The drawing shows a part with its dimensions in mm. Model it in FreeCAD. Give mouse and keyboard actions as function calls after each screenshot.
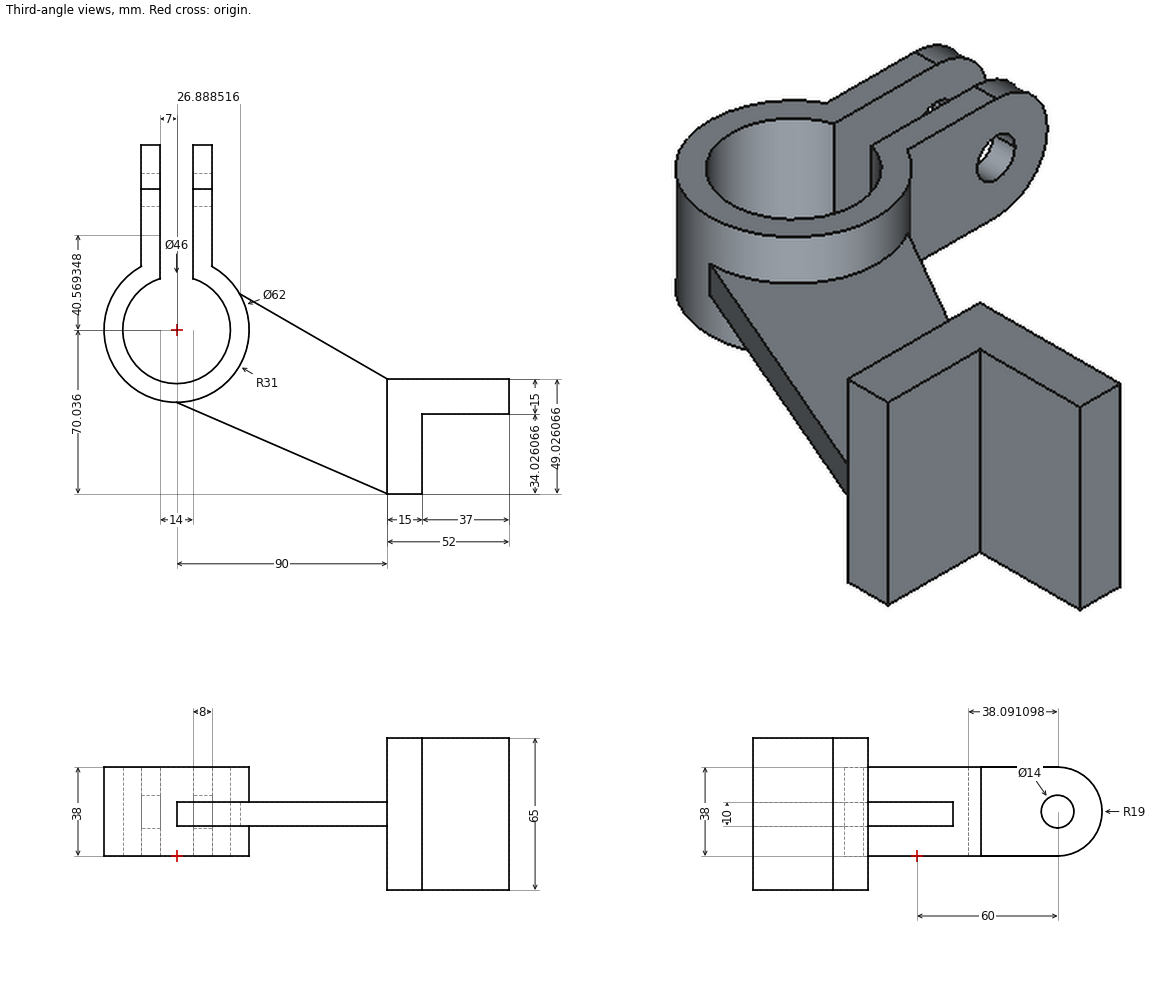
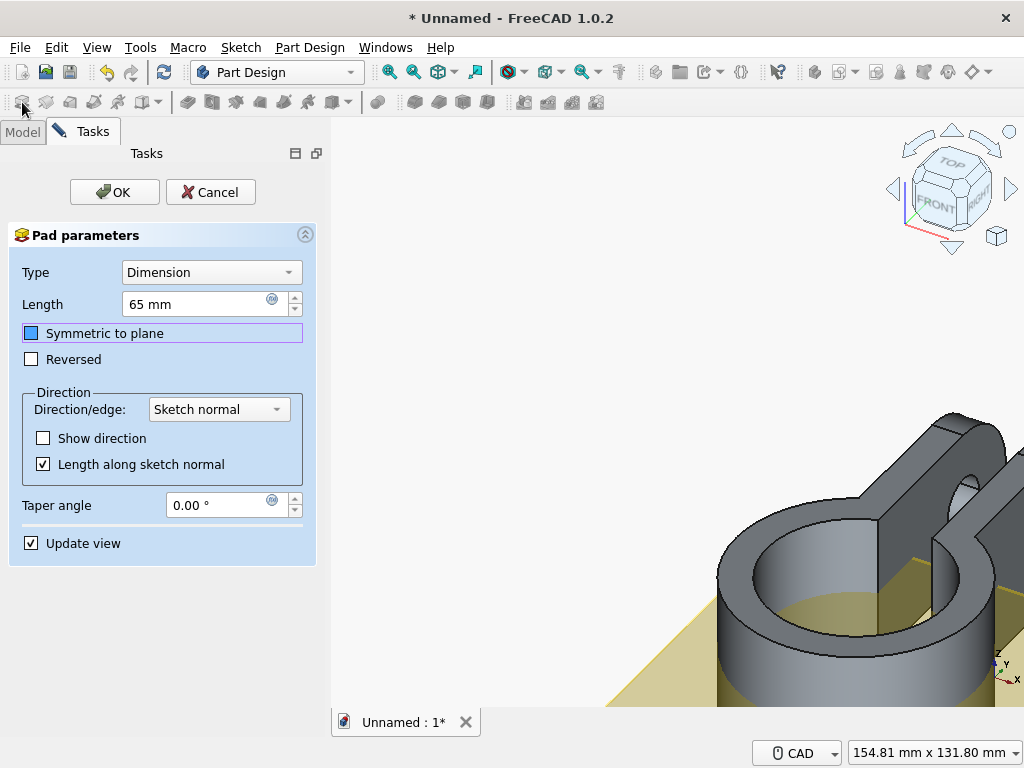
click(30, 333)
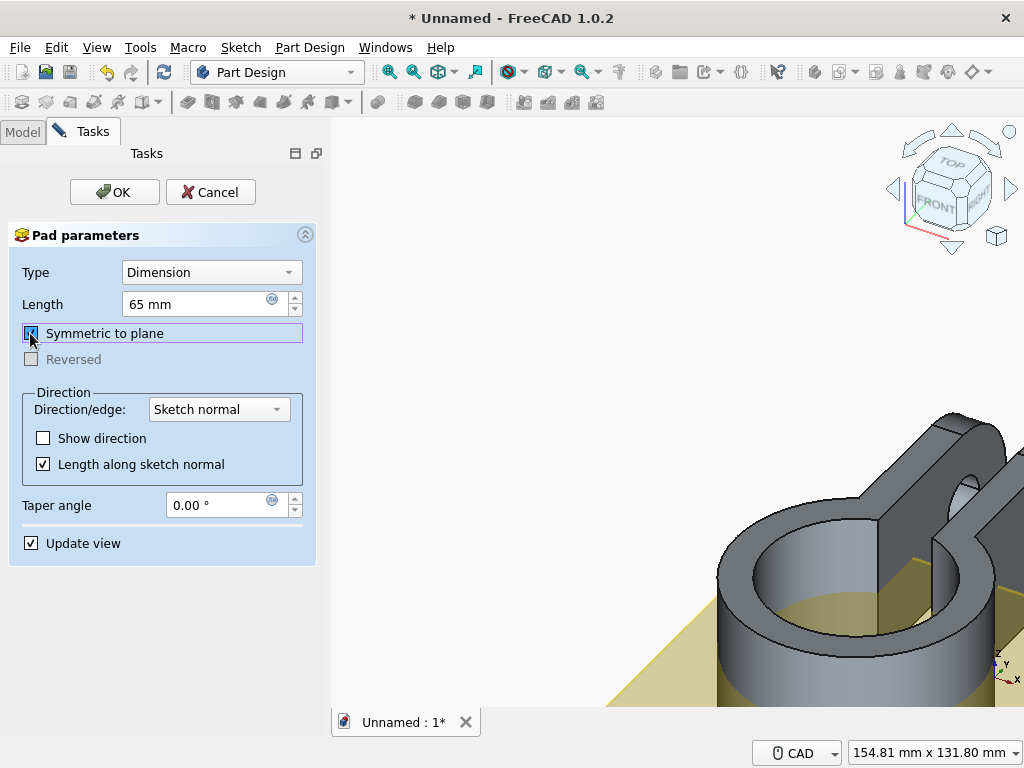
click(115, 192)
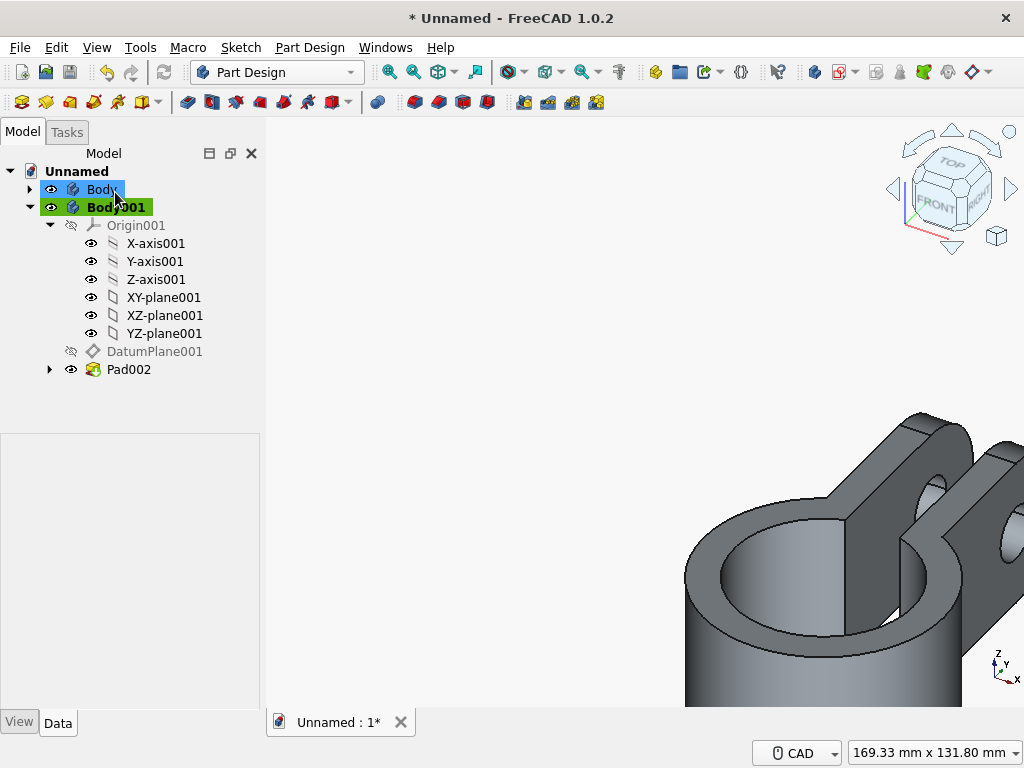
click(390, 72)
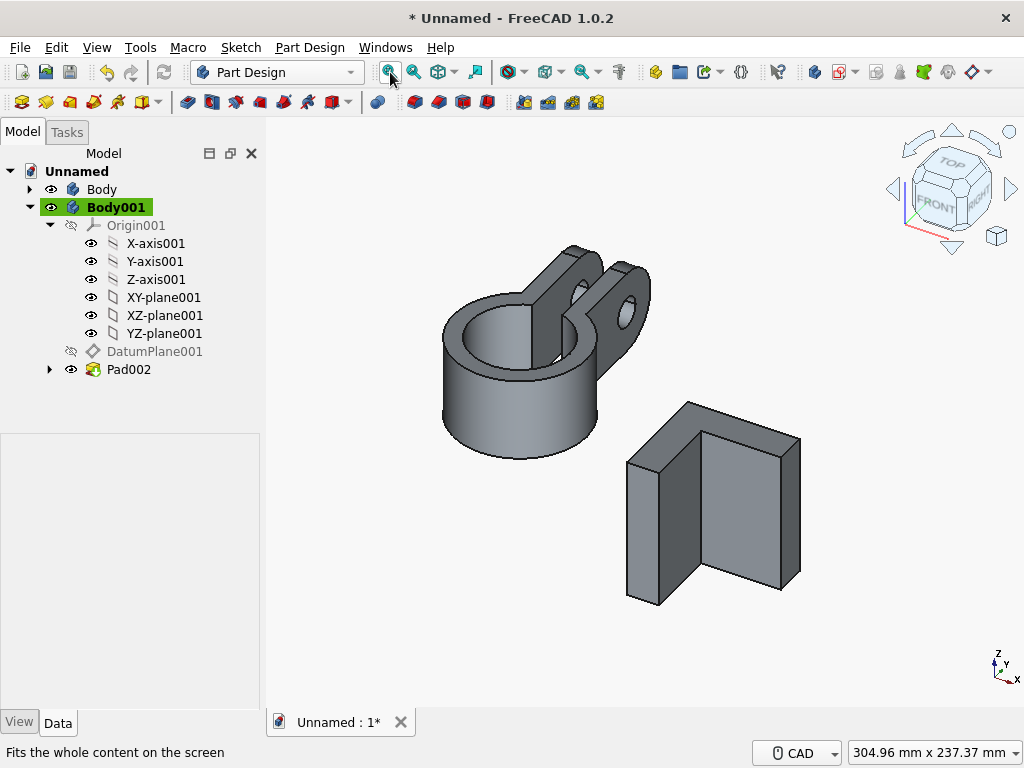
double_click(96, 189)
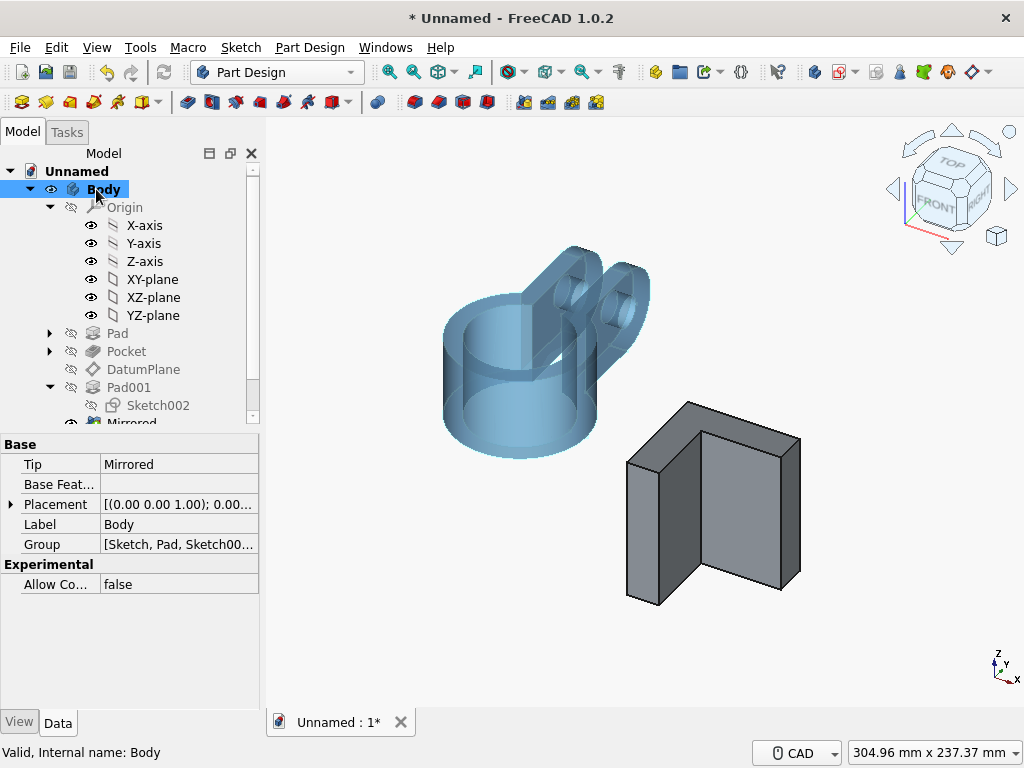
click(96, 189)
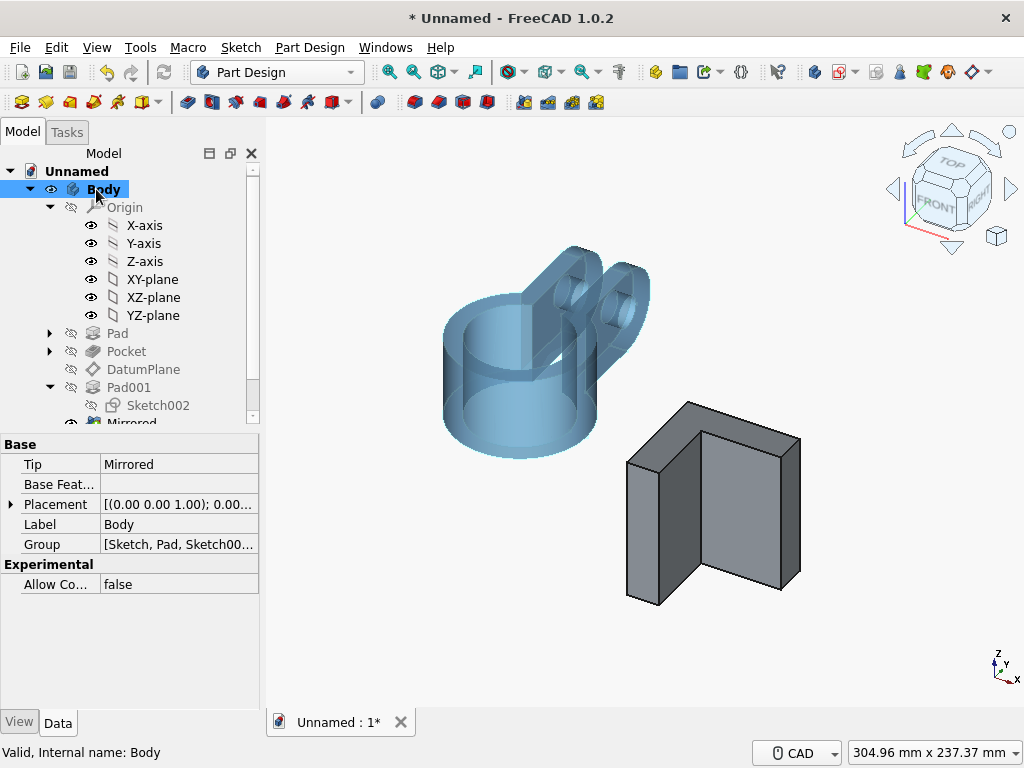
click(146, 584)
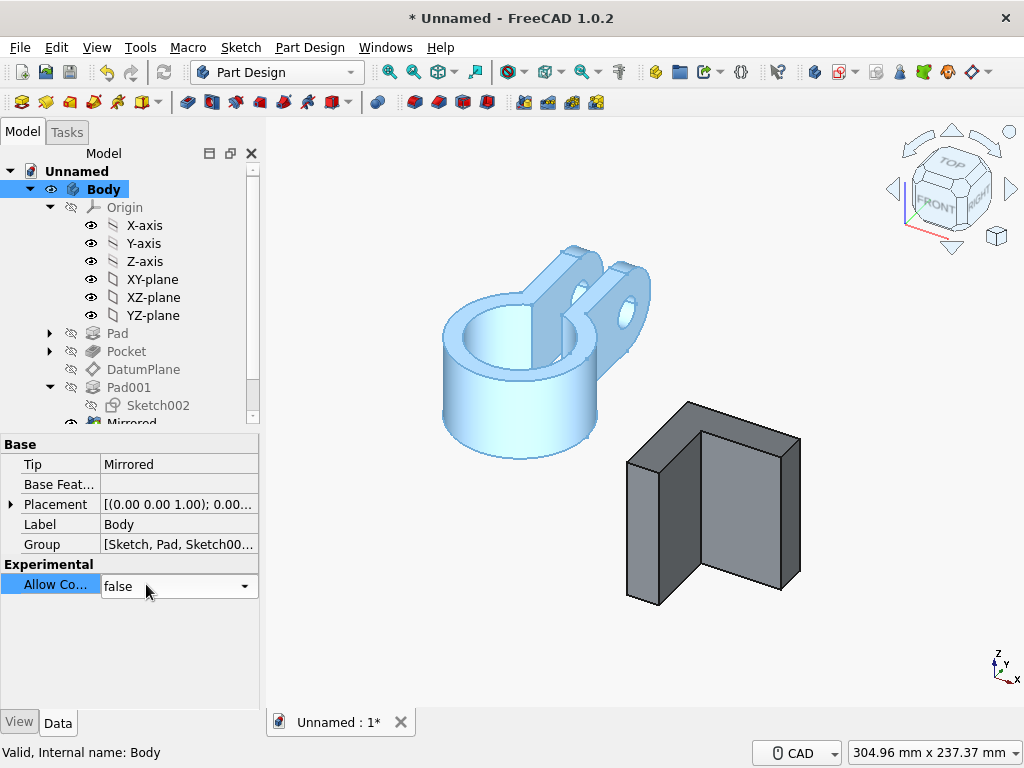
click(146, 584)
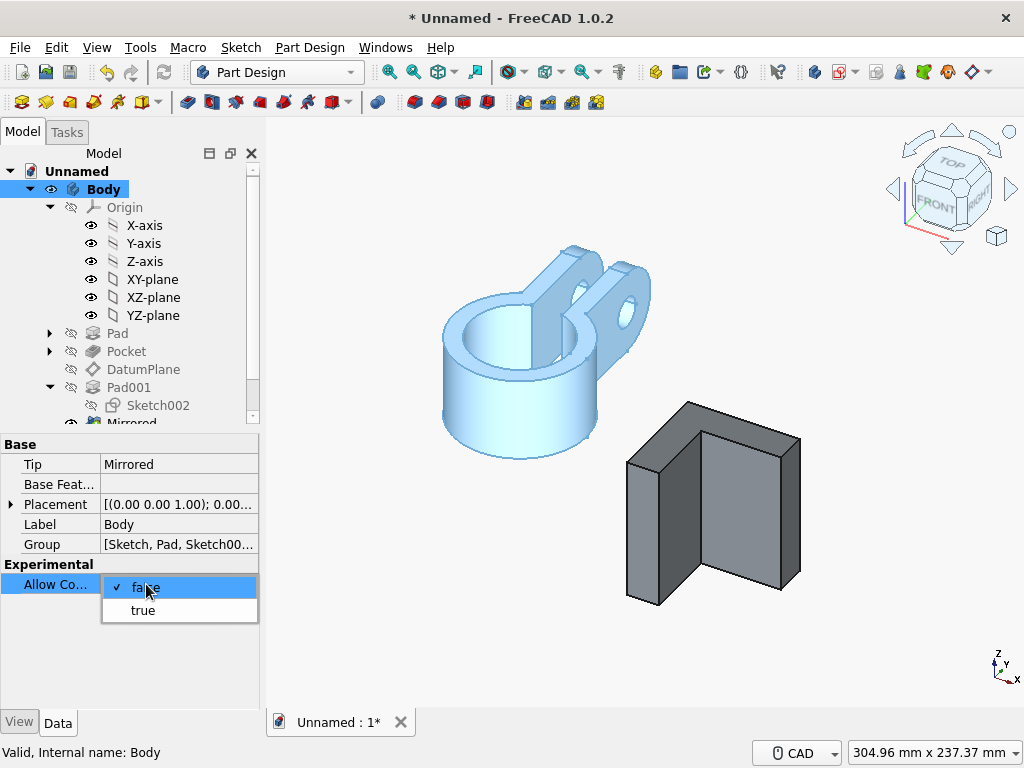
click(179, 610)
key(Return)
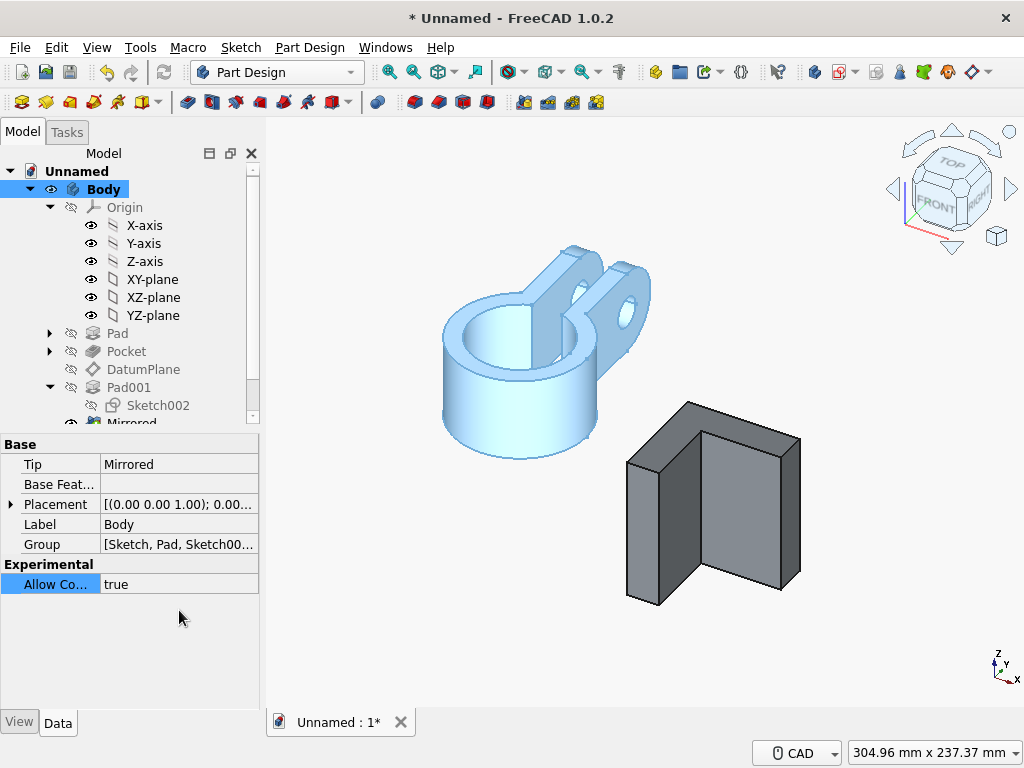
scroll(100, 293, down, 3)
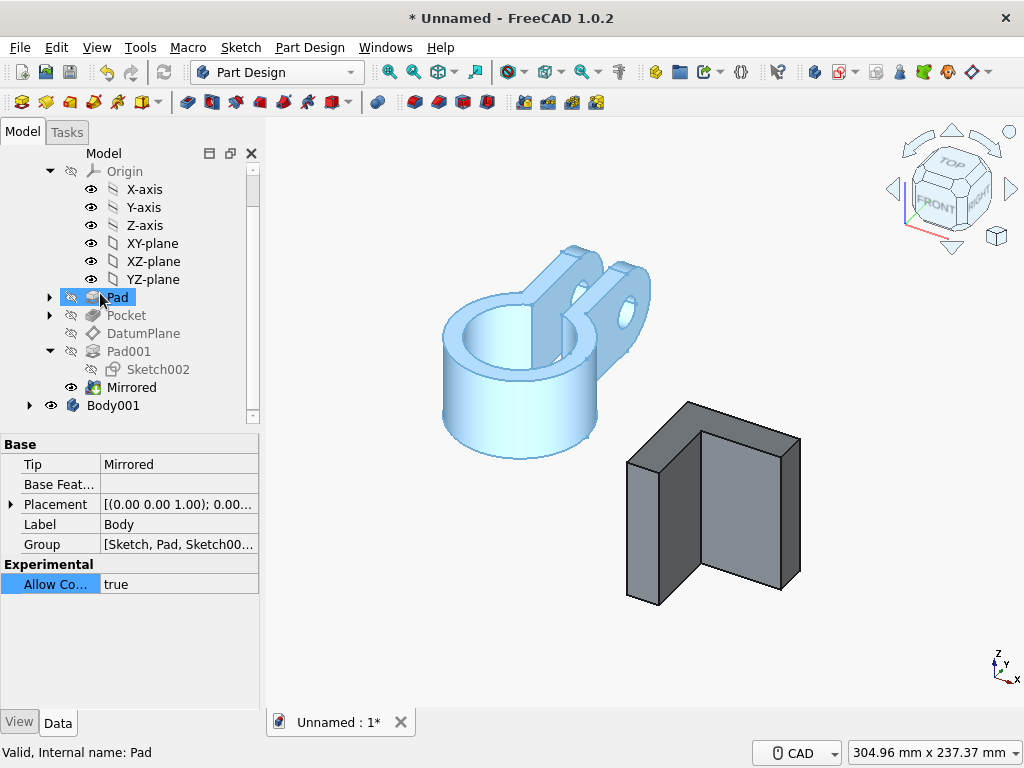
click(96, 405)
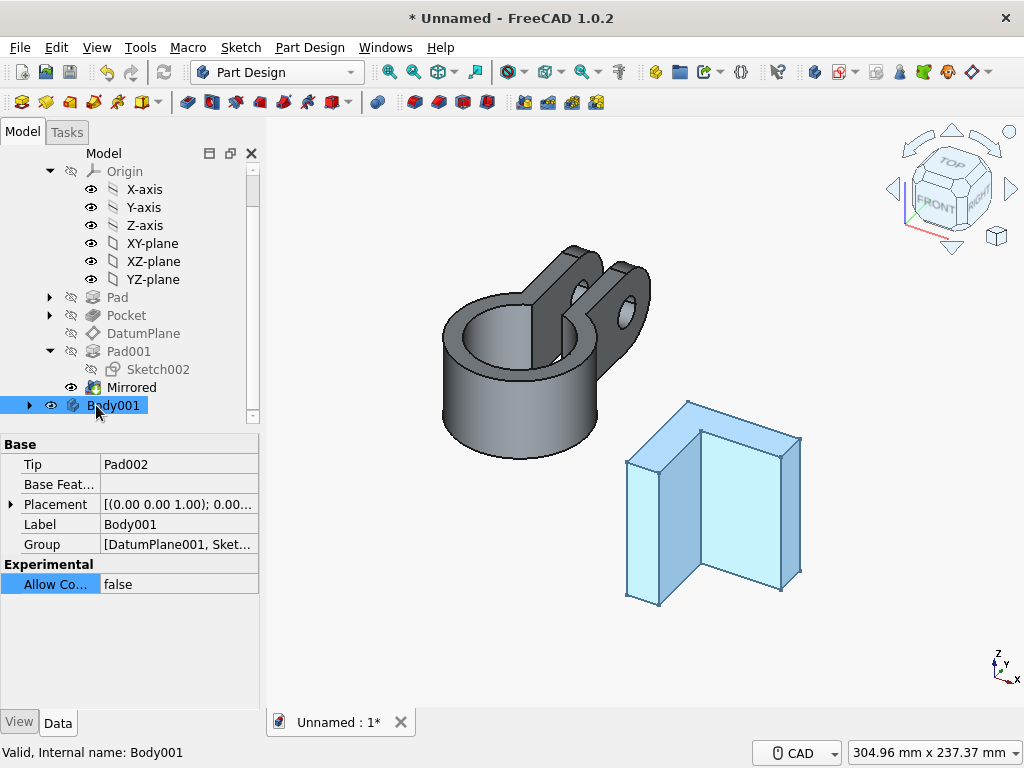
click(378, 102)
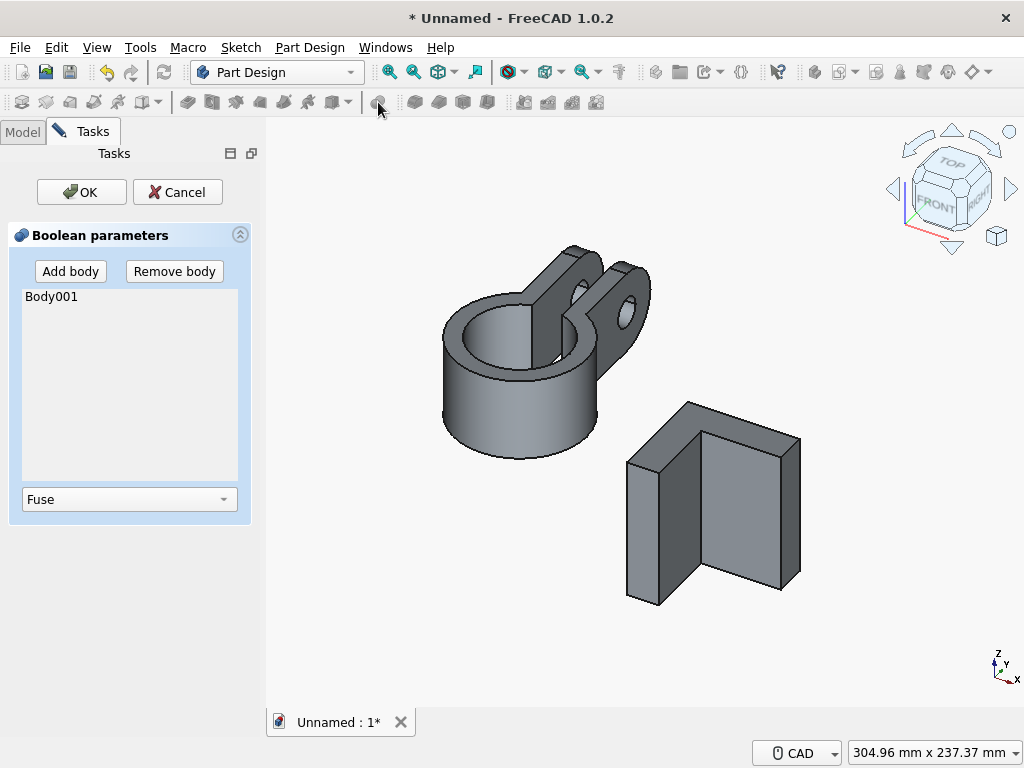
click(82, 192)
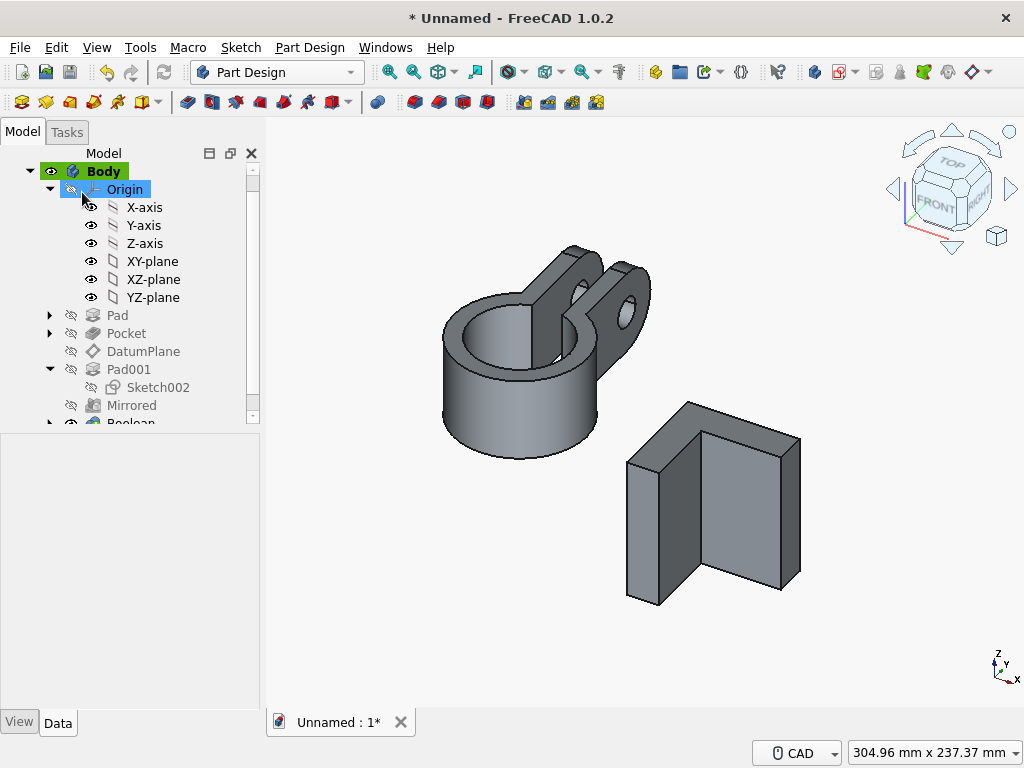
click(136, 261)